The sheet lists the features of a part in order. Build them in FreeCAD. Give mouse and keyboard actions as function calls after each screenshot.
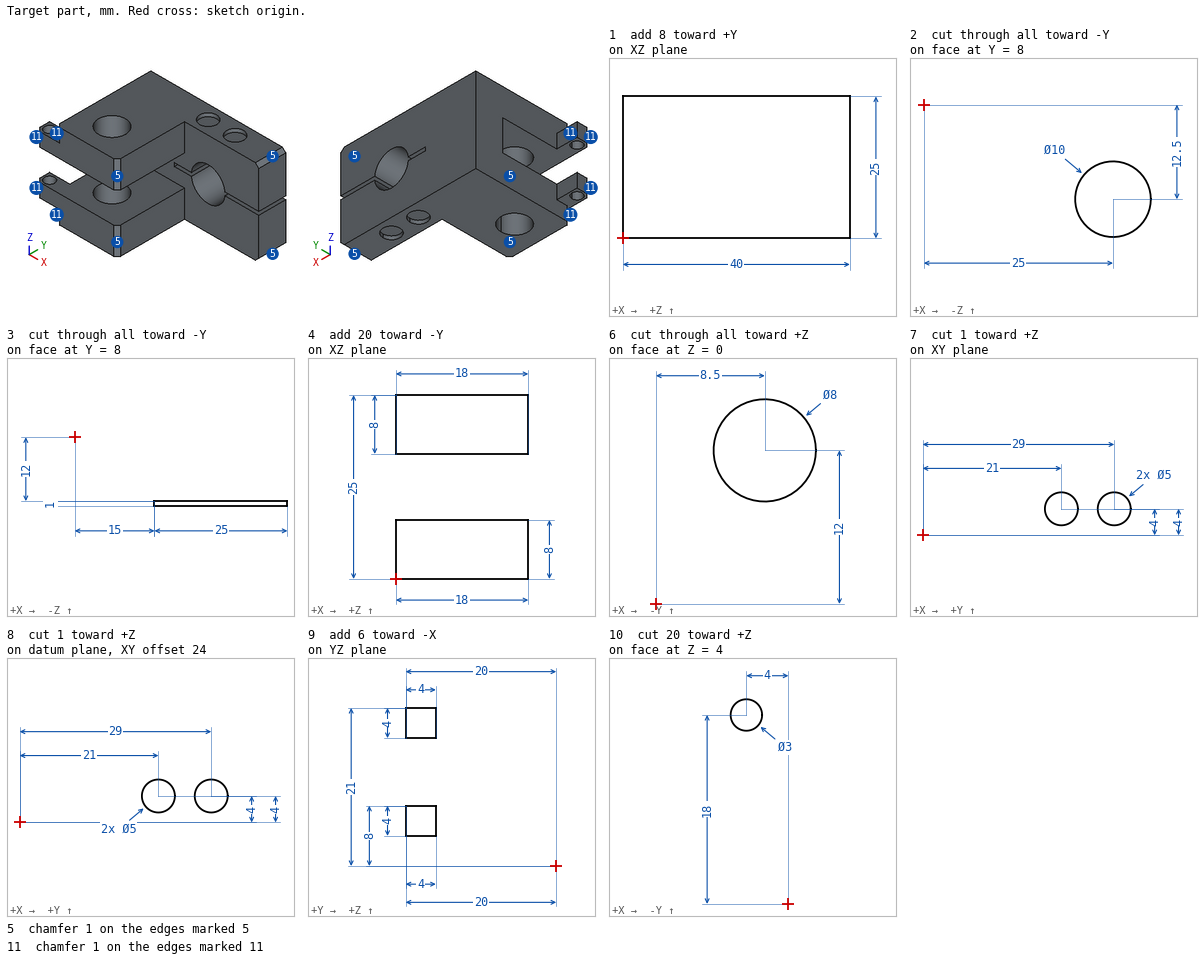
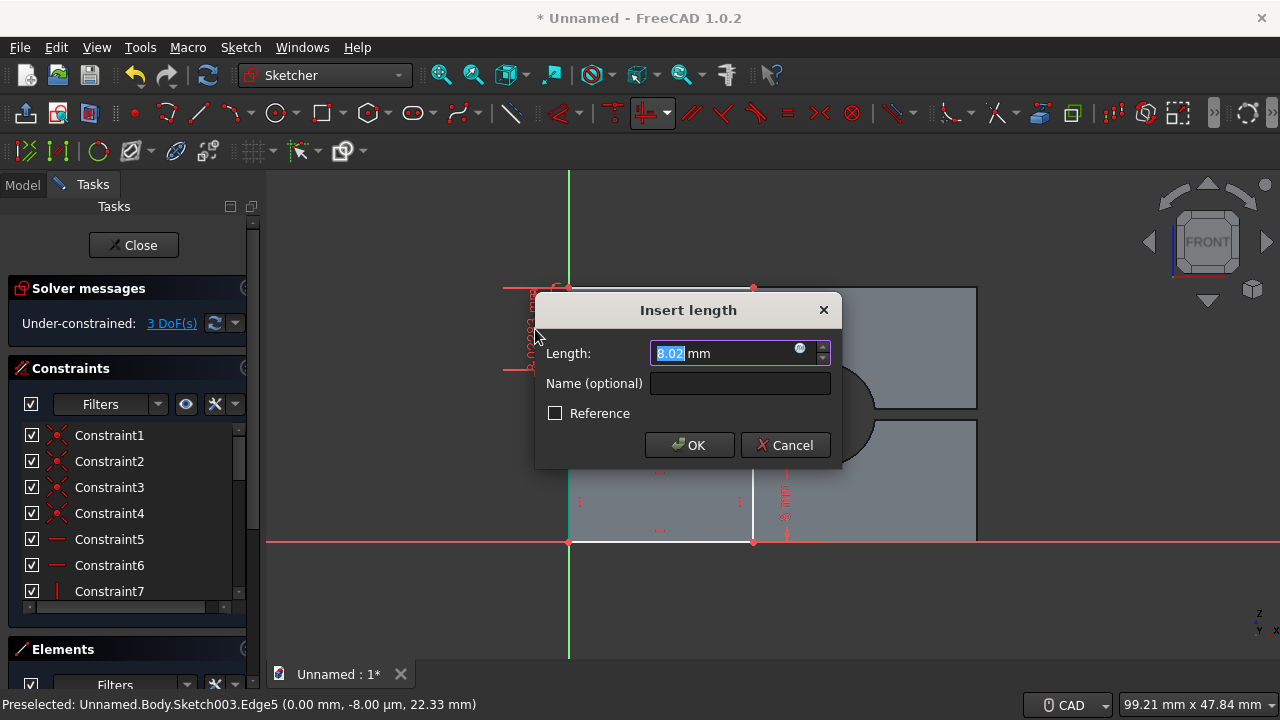
text(8)
key(Return)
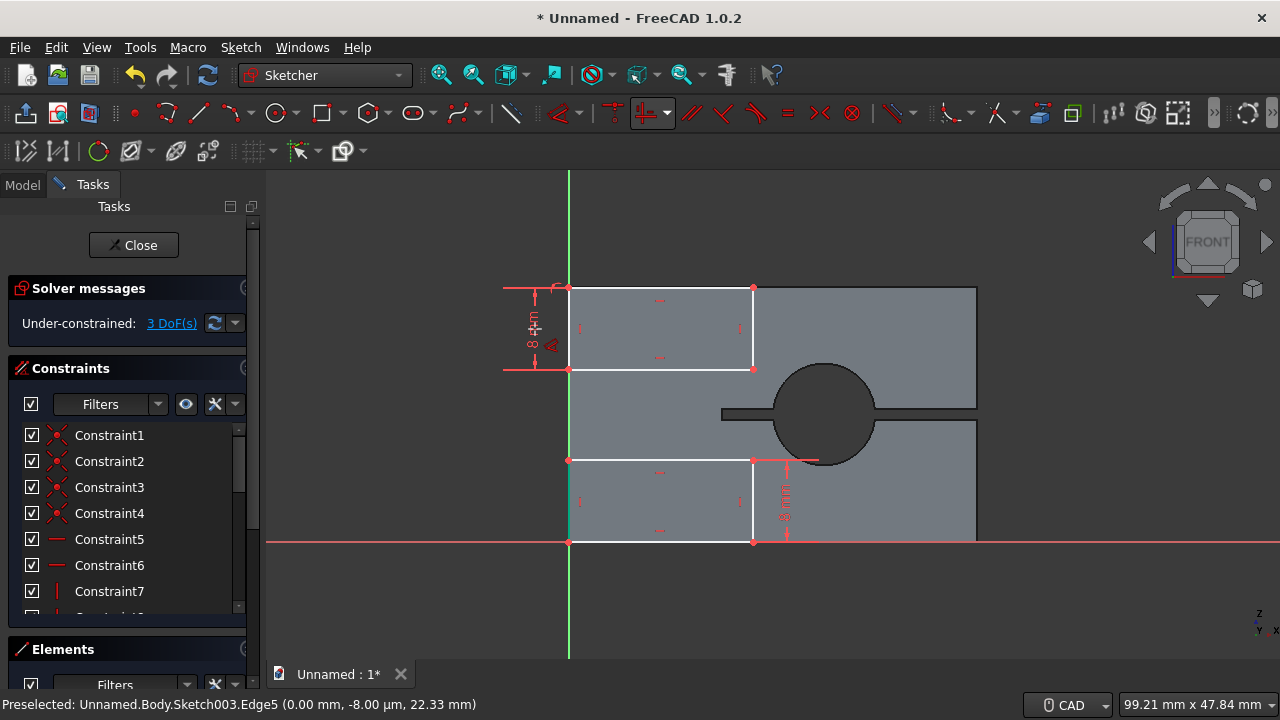
click(624, 542)
click(661, 576)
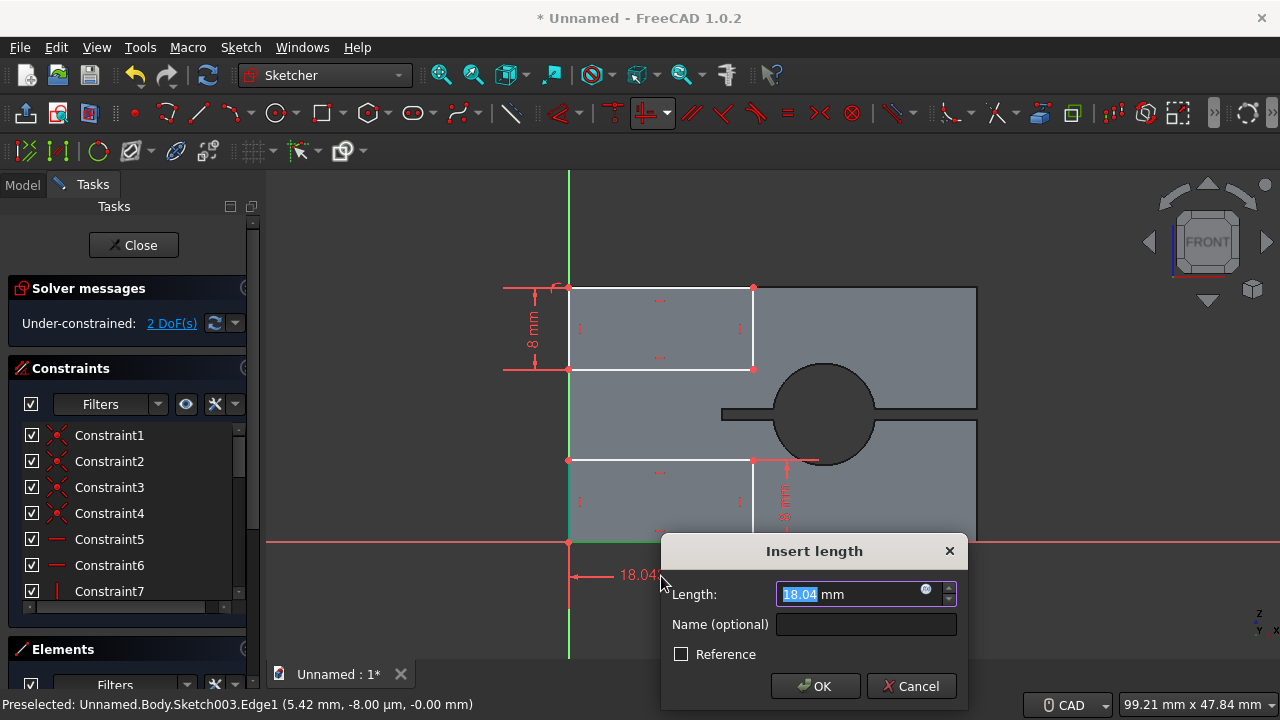
text(18)
key(Return)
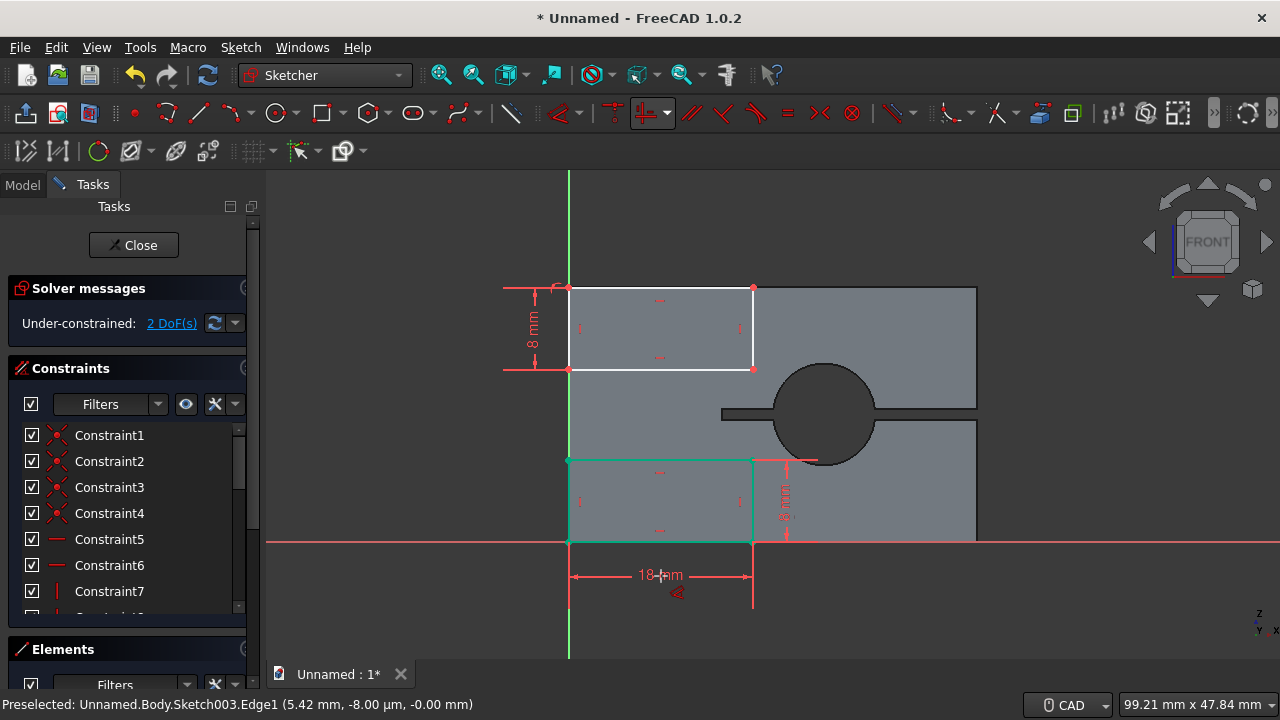
click(624, 370)
click(661, 336)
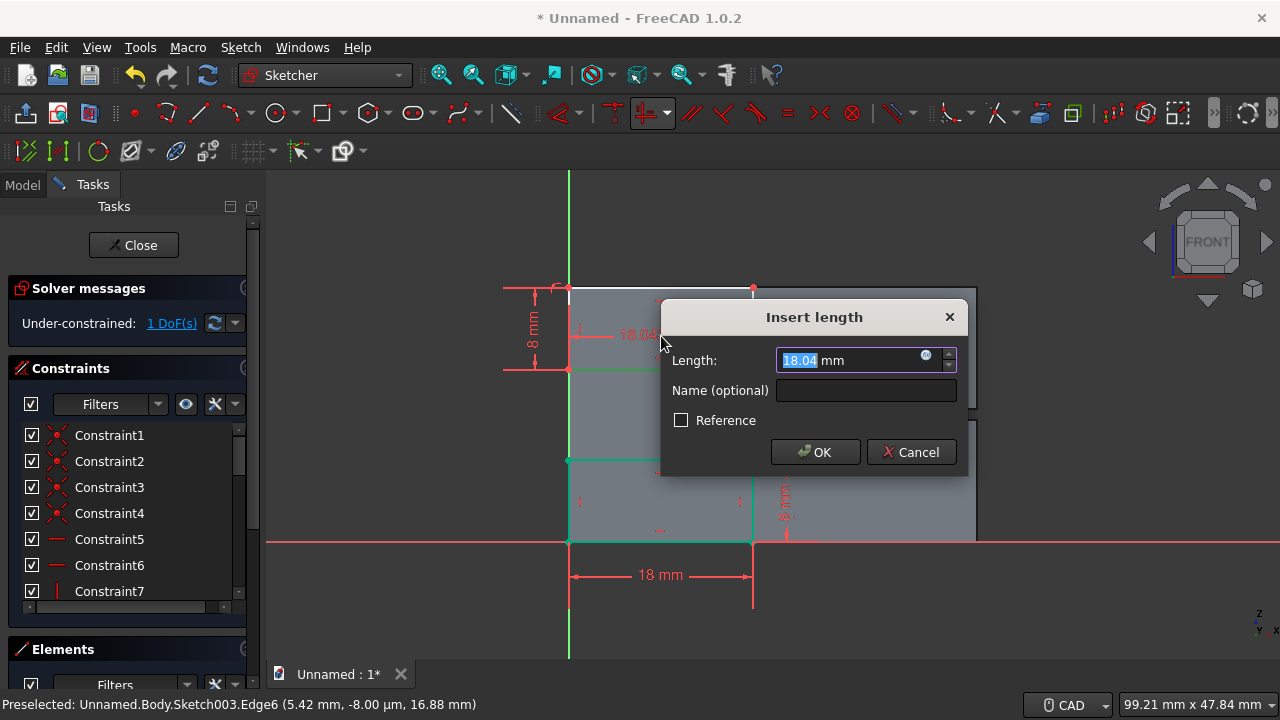
text(18)
key(Return)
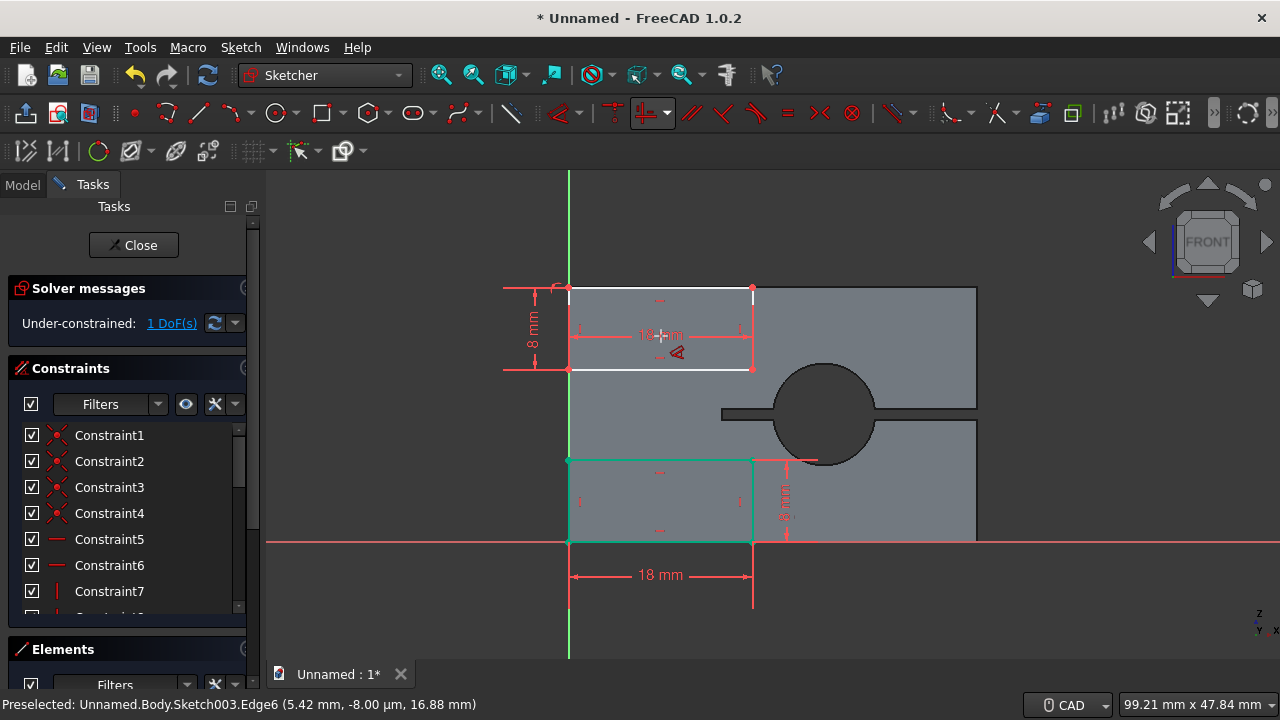
click(569, 288)
click(535, 415)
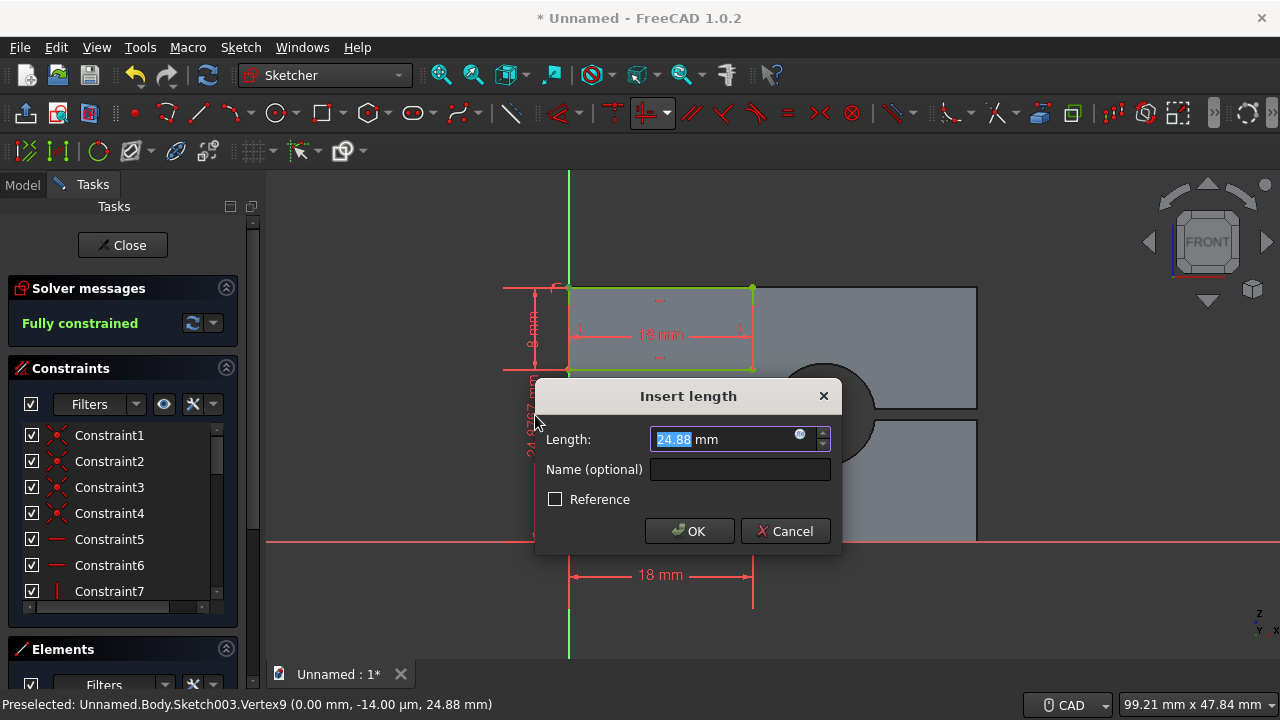
text(25)
key(Return)
key(Escape)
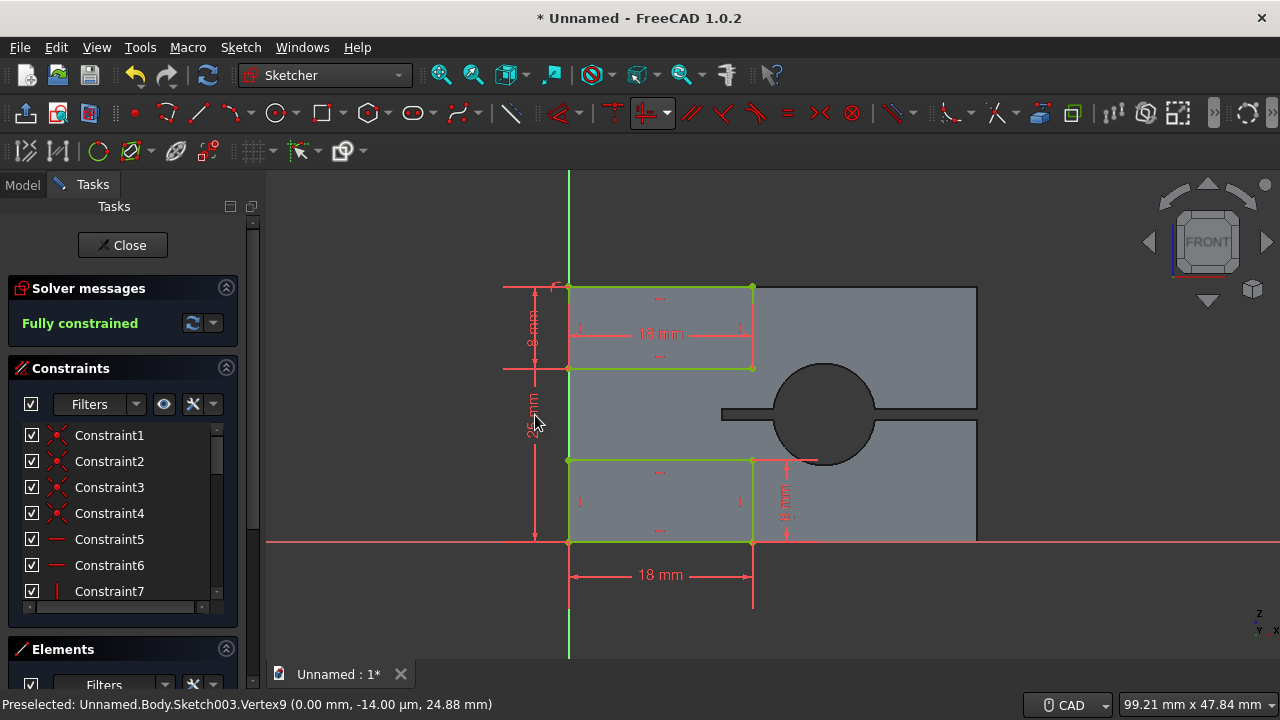
click(123, 245)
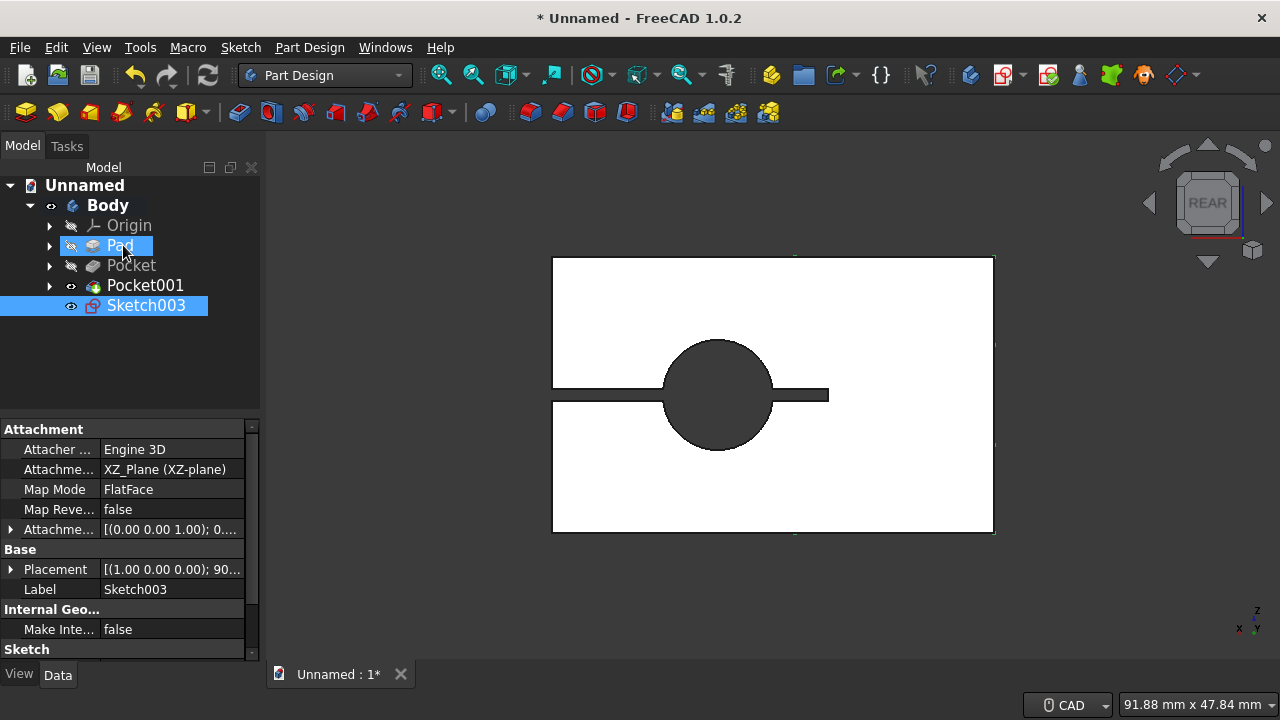
click(26, 112)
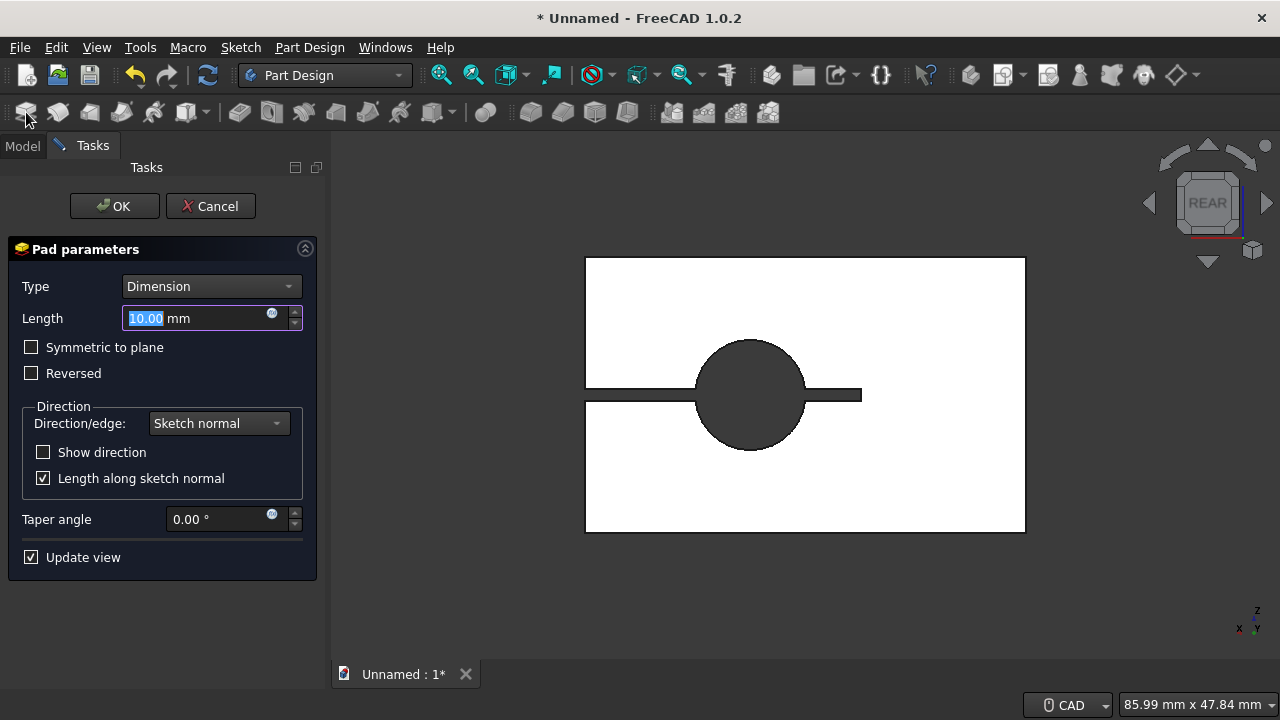
text(20)
key(Tab)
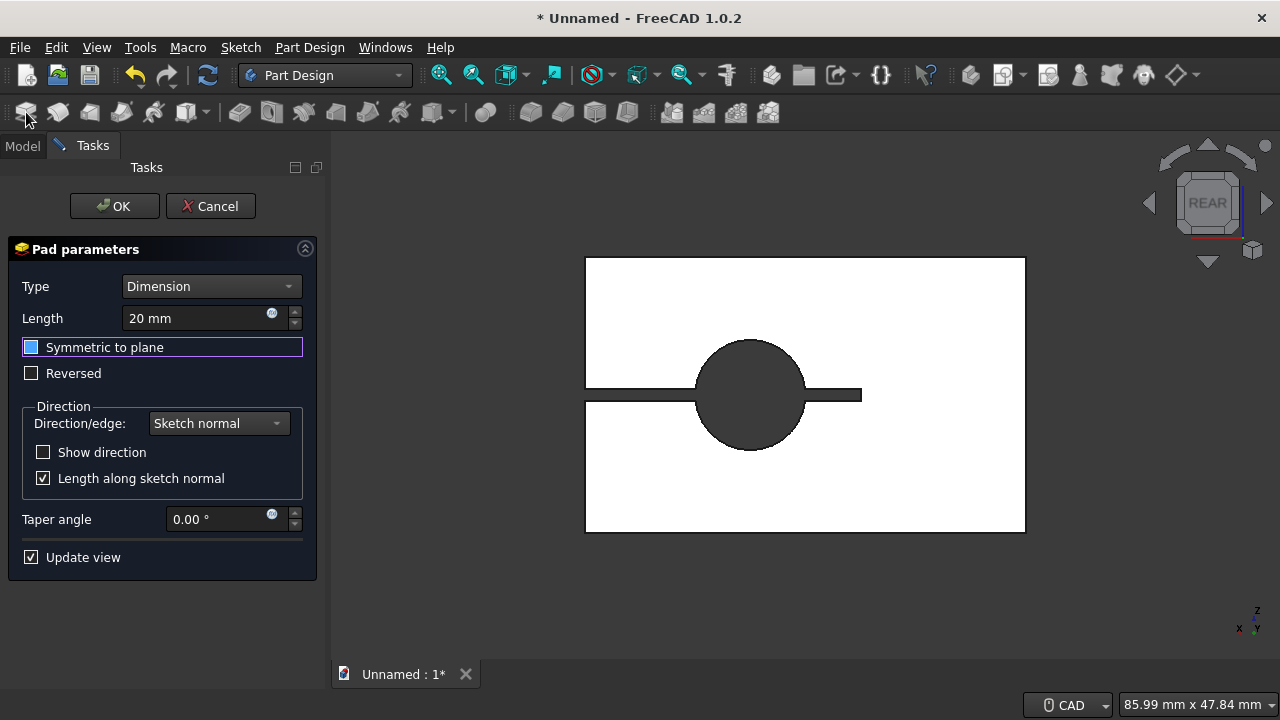
click(115, 206)